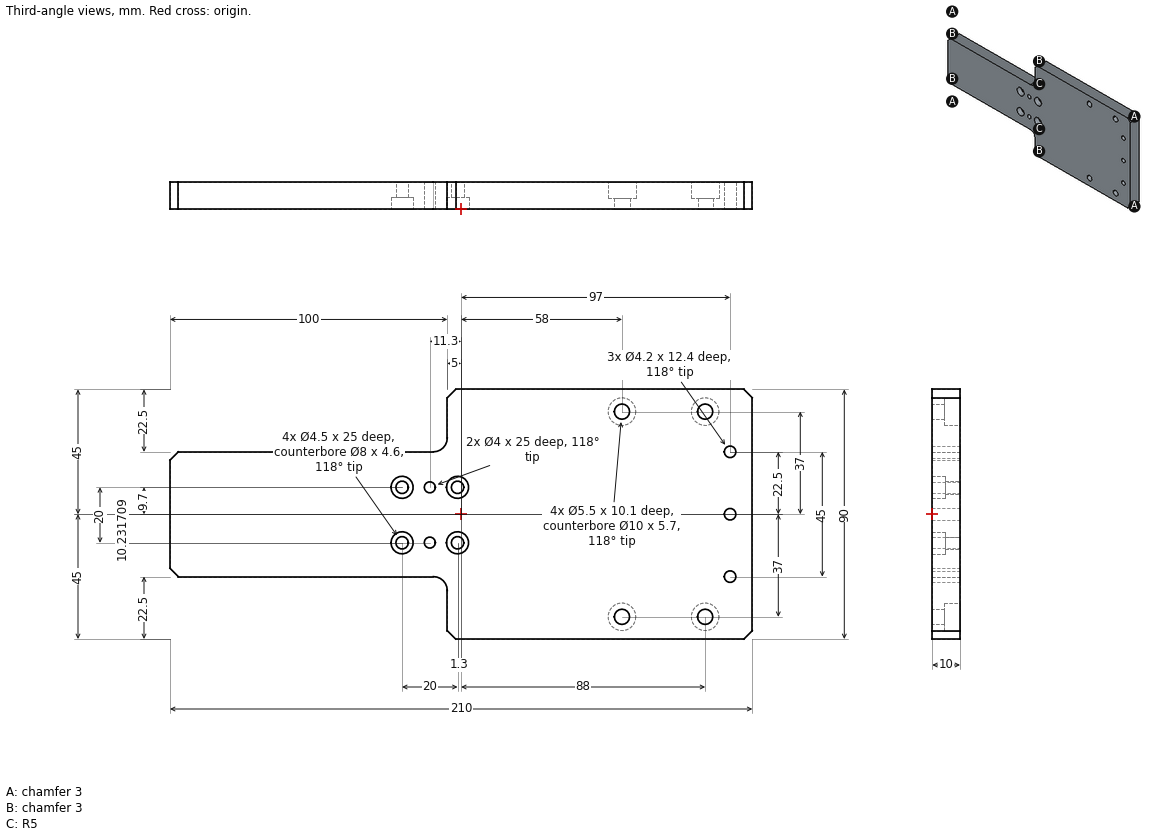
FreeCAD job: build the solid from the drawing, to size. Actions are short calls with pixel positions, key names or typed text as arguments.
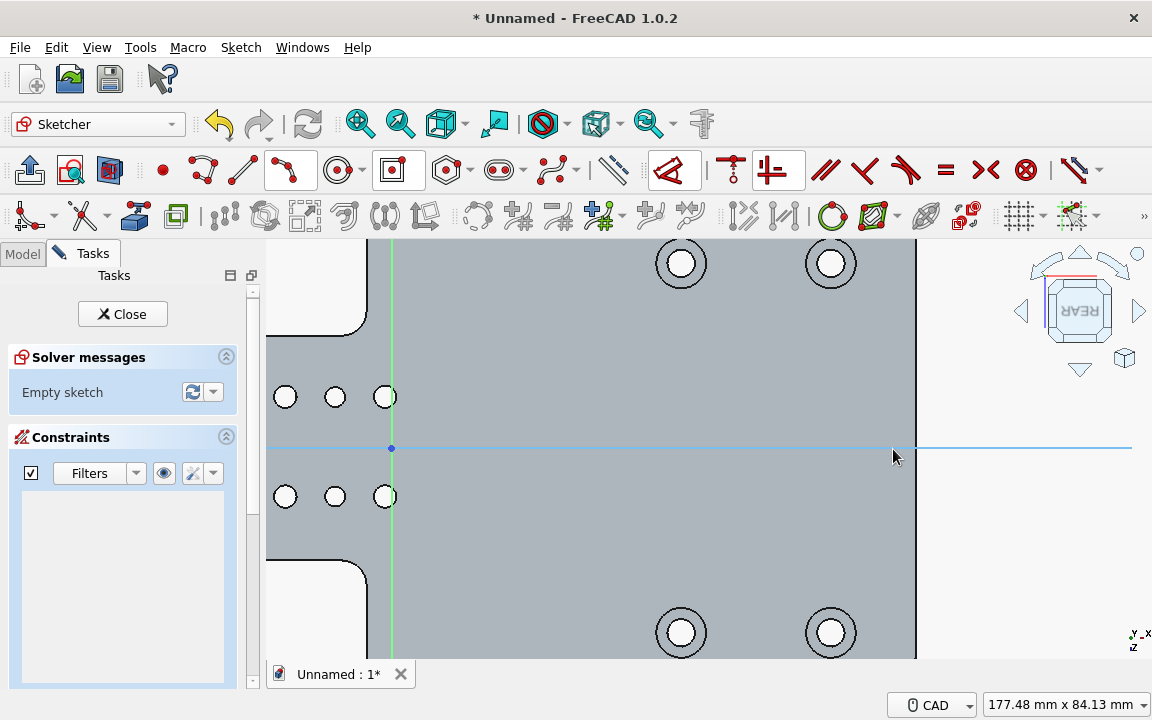
click(338, 170)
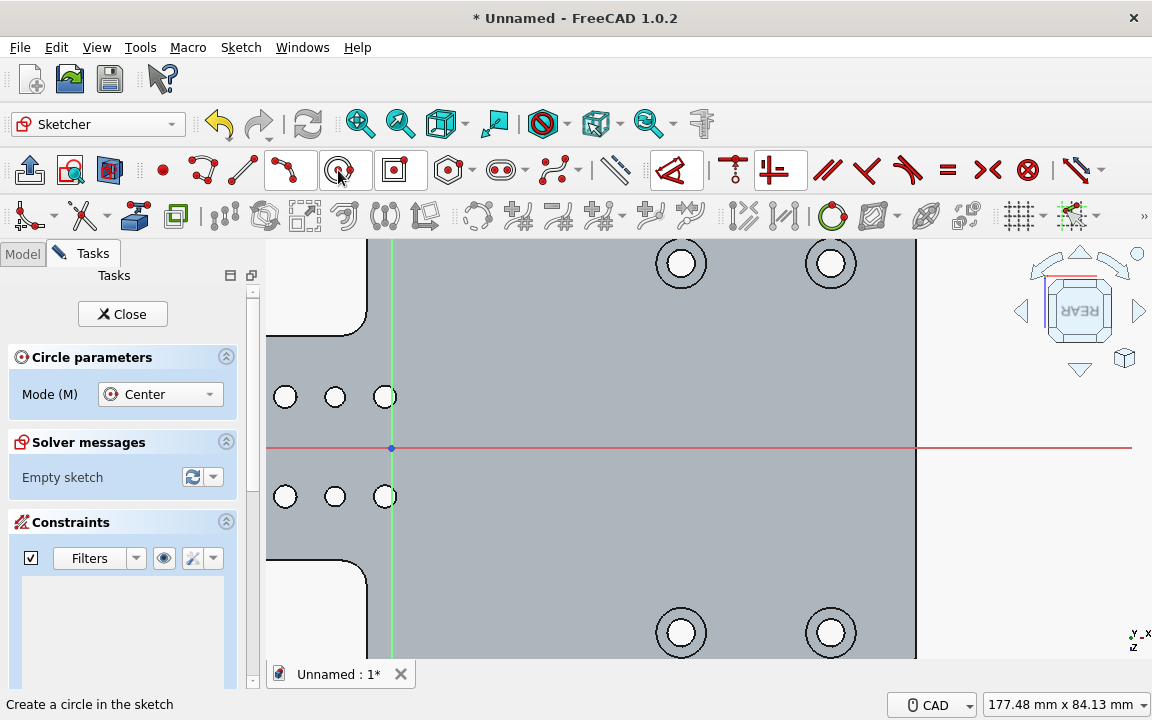
scroll(876, 560, up, 4)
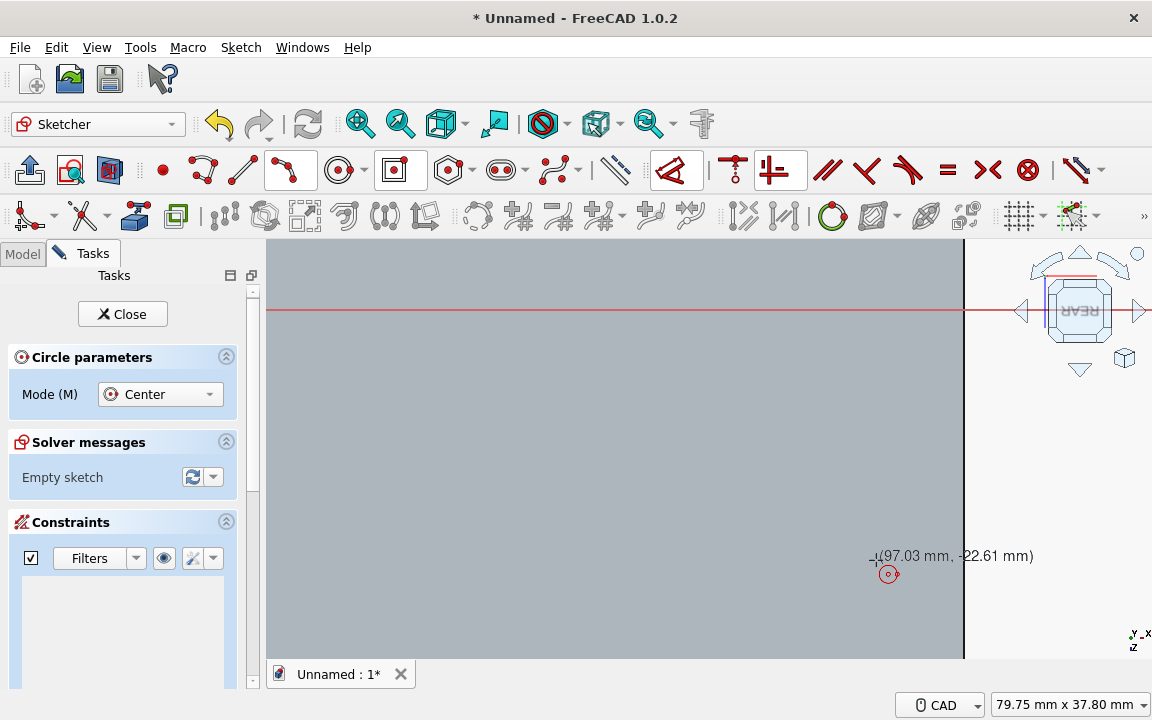
click(875, 560)
click(891, 544)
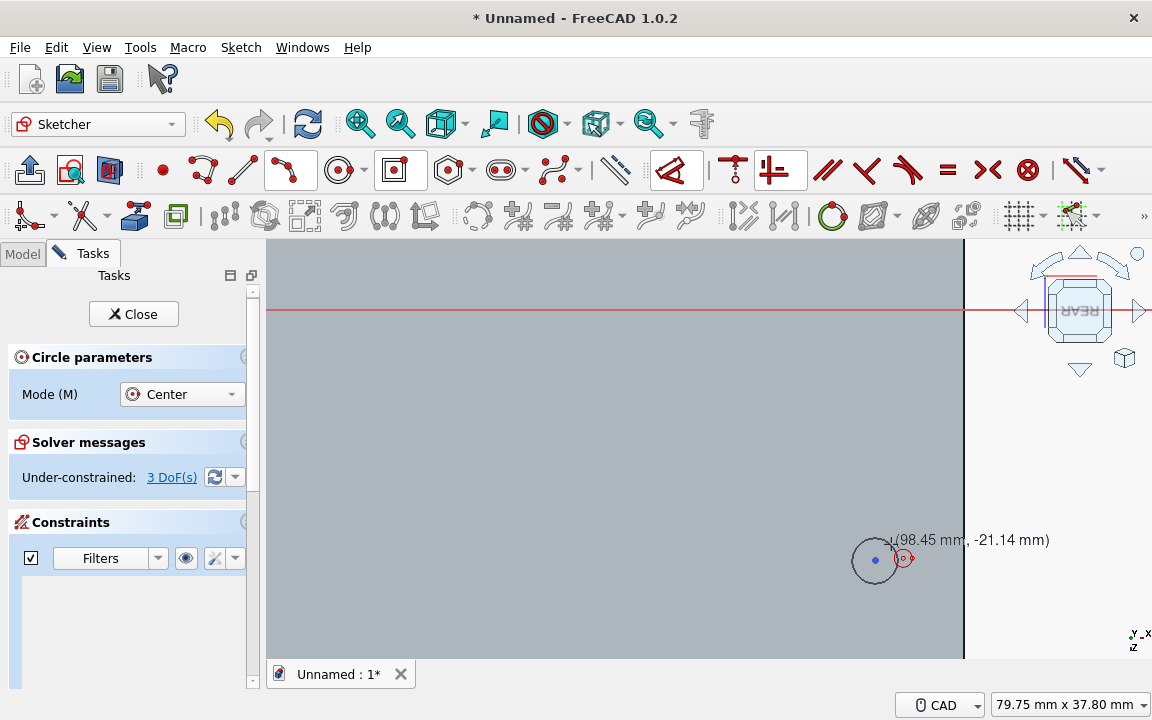
click(875, 310)
click(891, 294)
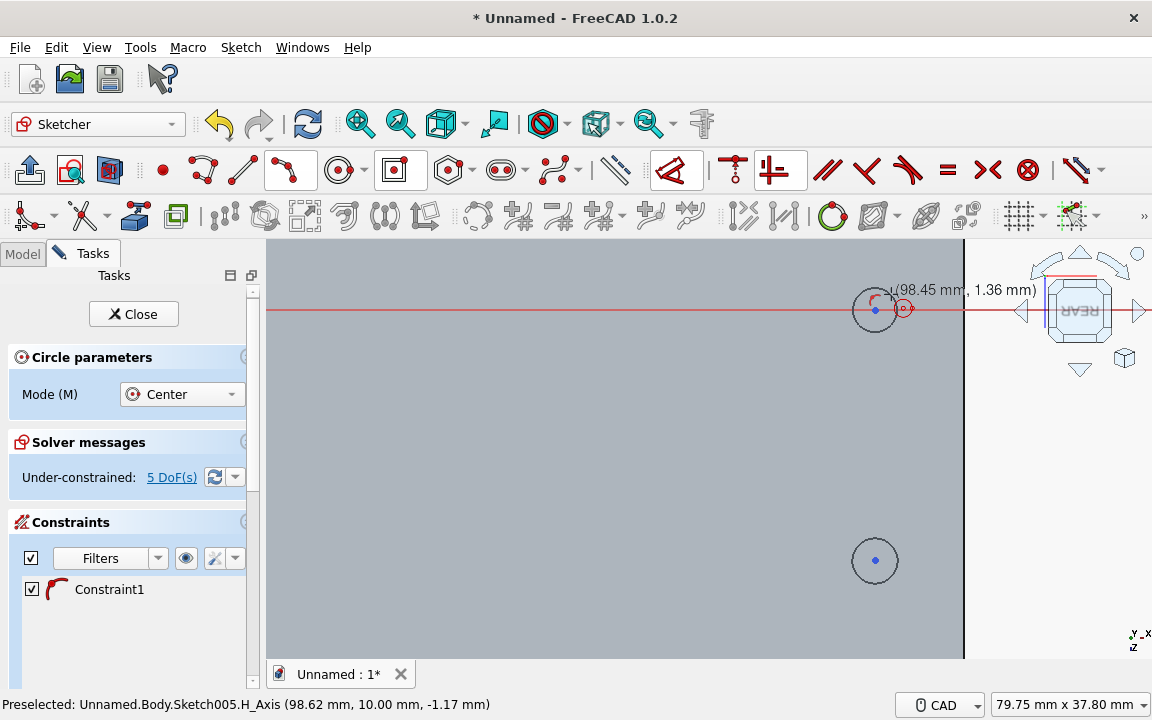
scroll(879, 562, down, 4)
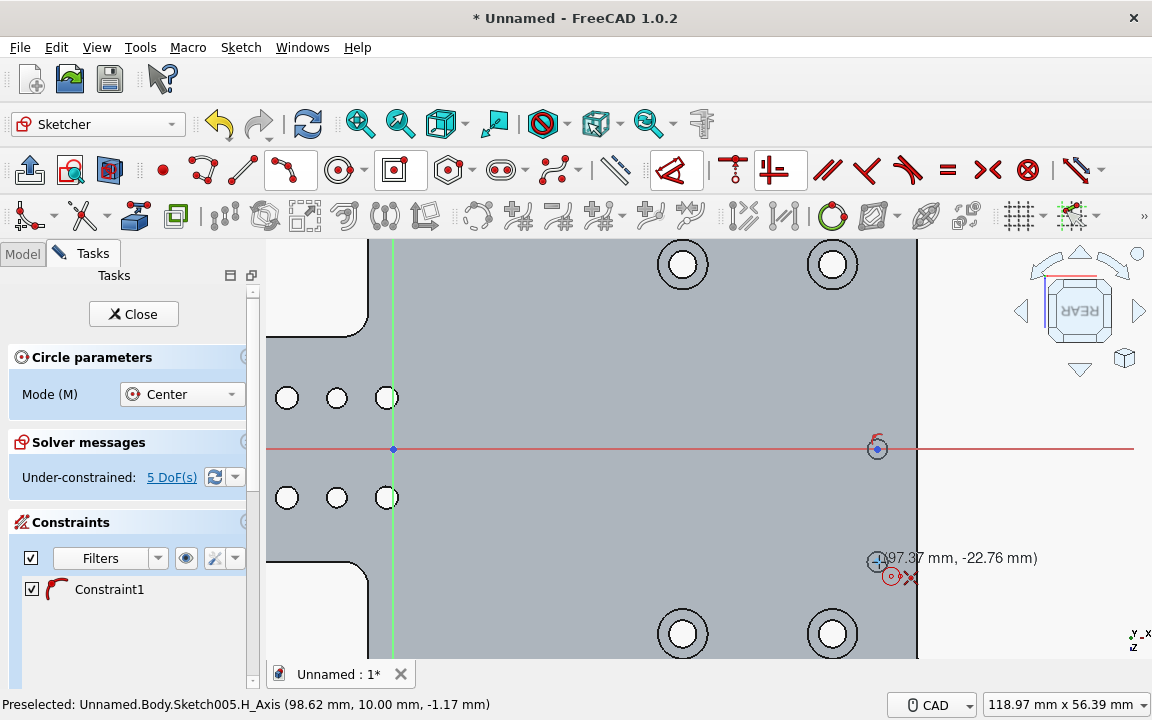
scroll(878, 337, up, 4)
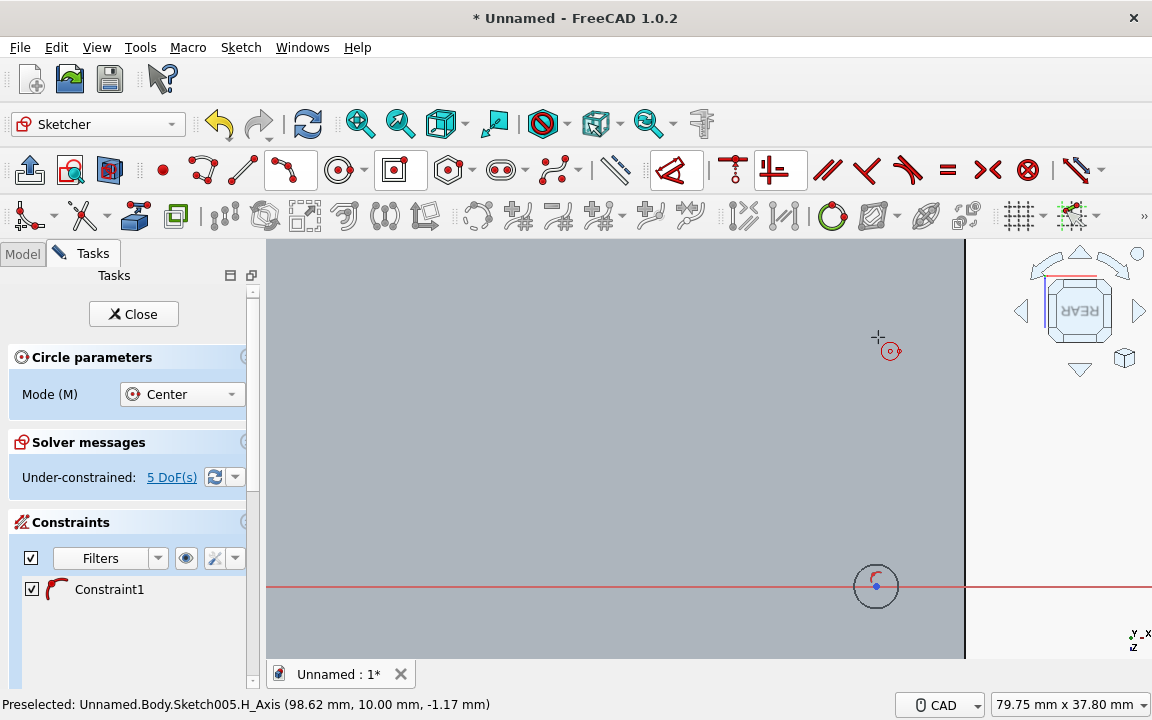
click(876, 337)
click(893, 320)
key(Escape)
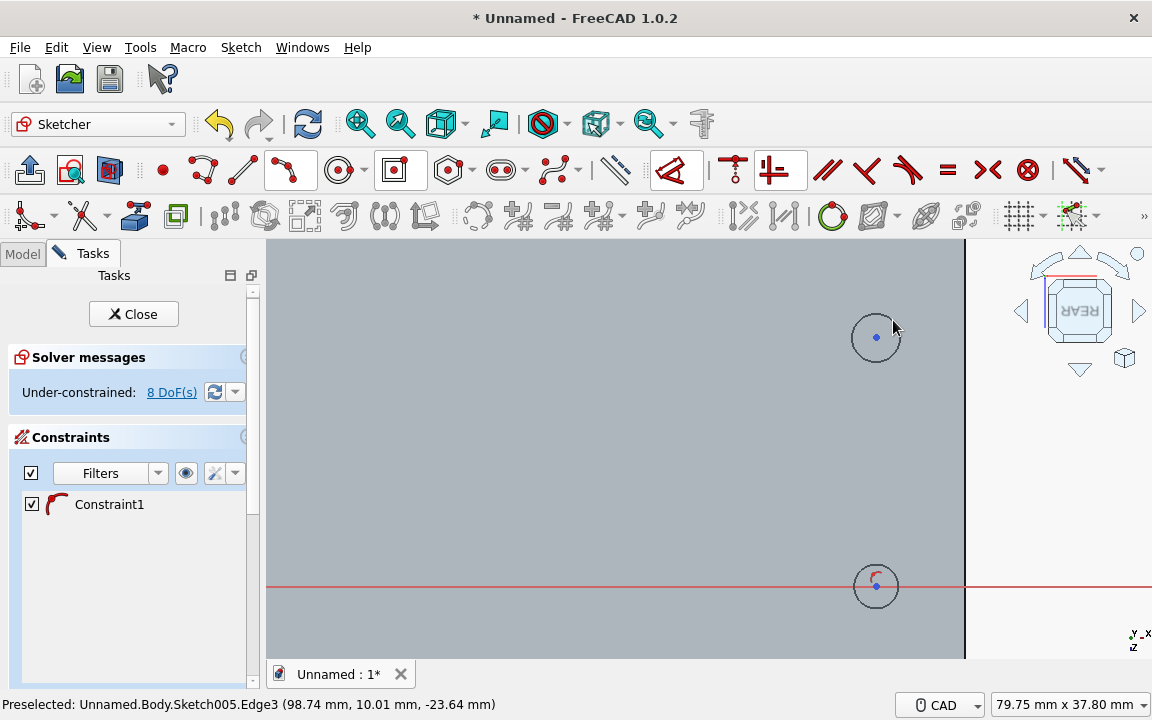
scroll(878, 337, down, 4)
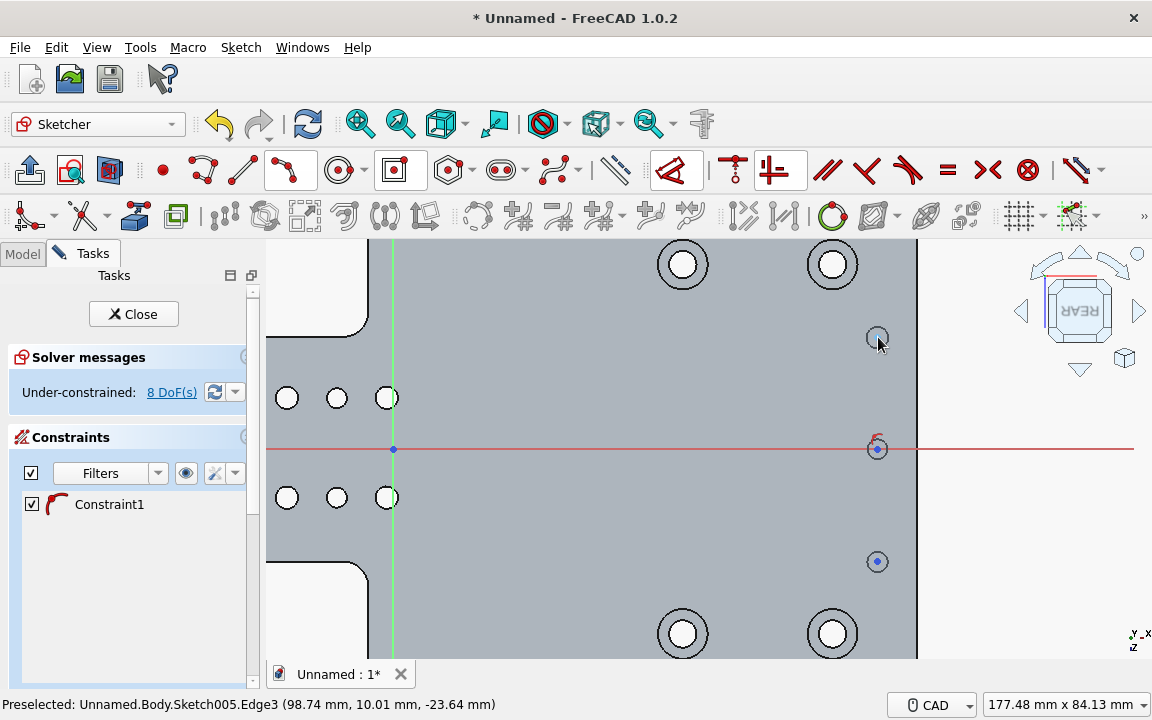
scroll(885, 555, up, 2)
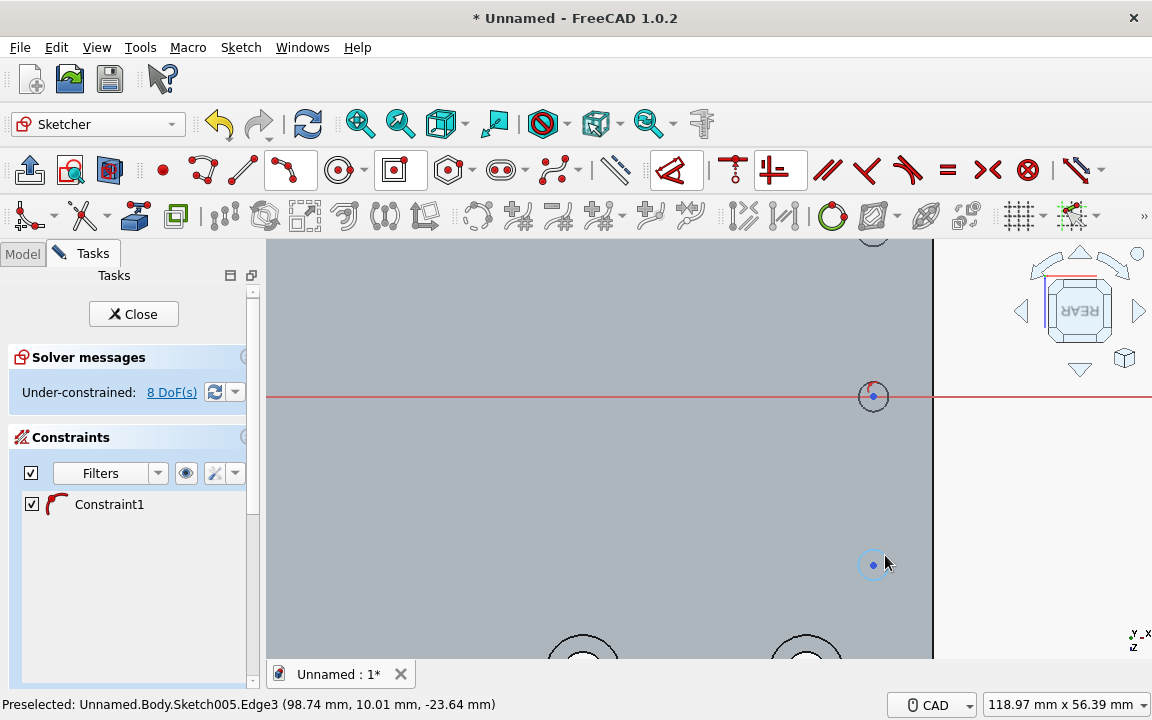
click(884, 554)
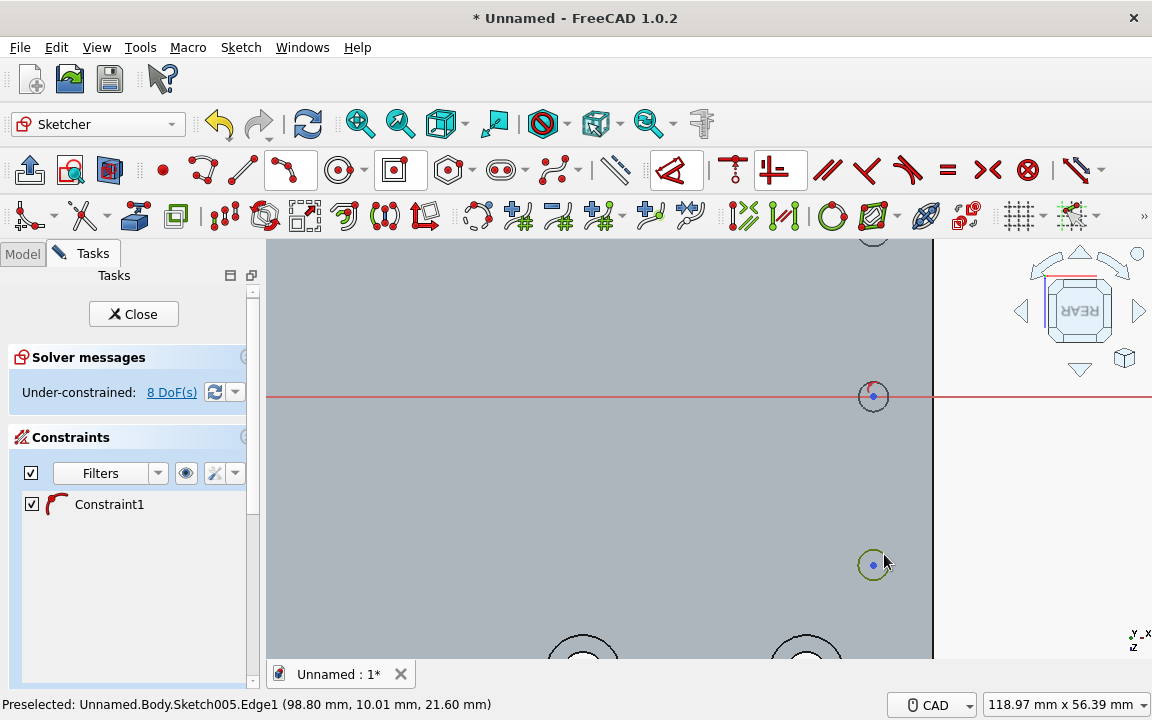
scroll(884, 386, up, 2)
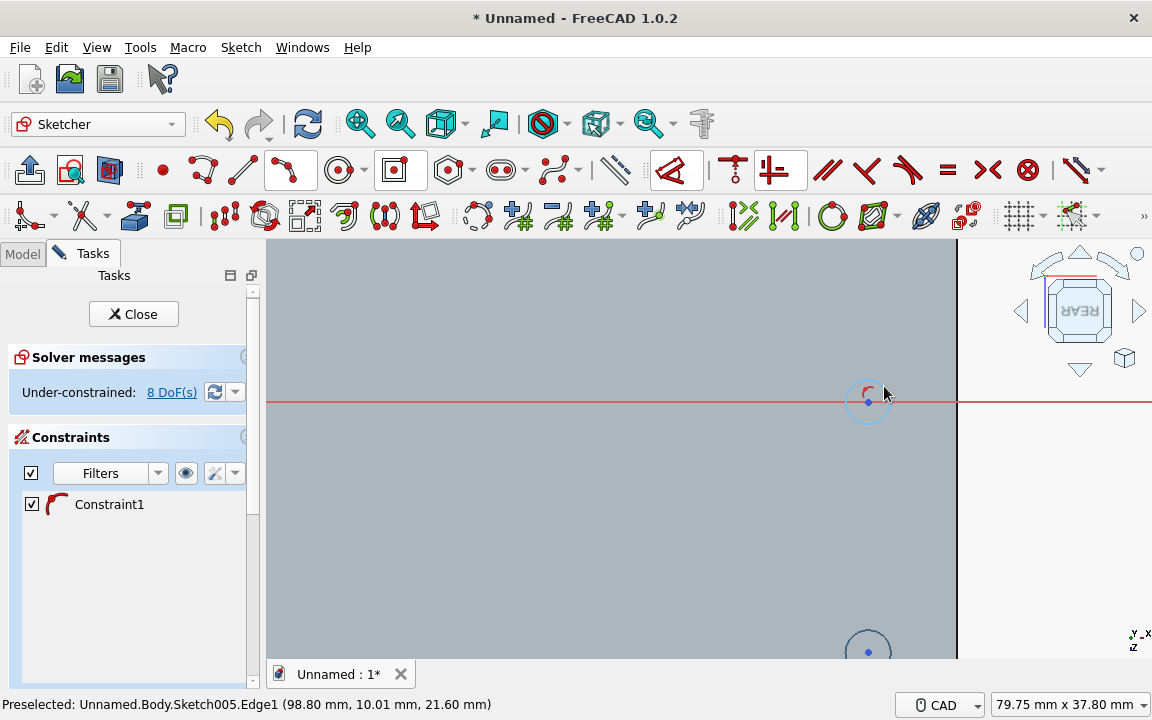
click(884, 386)